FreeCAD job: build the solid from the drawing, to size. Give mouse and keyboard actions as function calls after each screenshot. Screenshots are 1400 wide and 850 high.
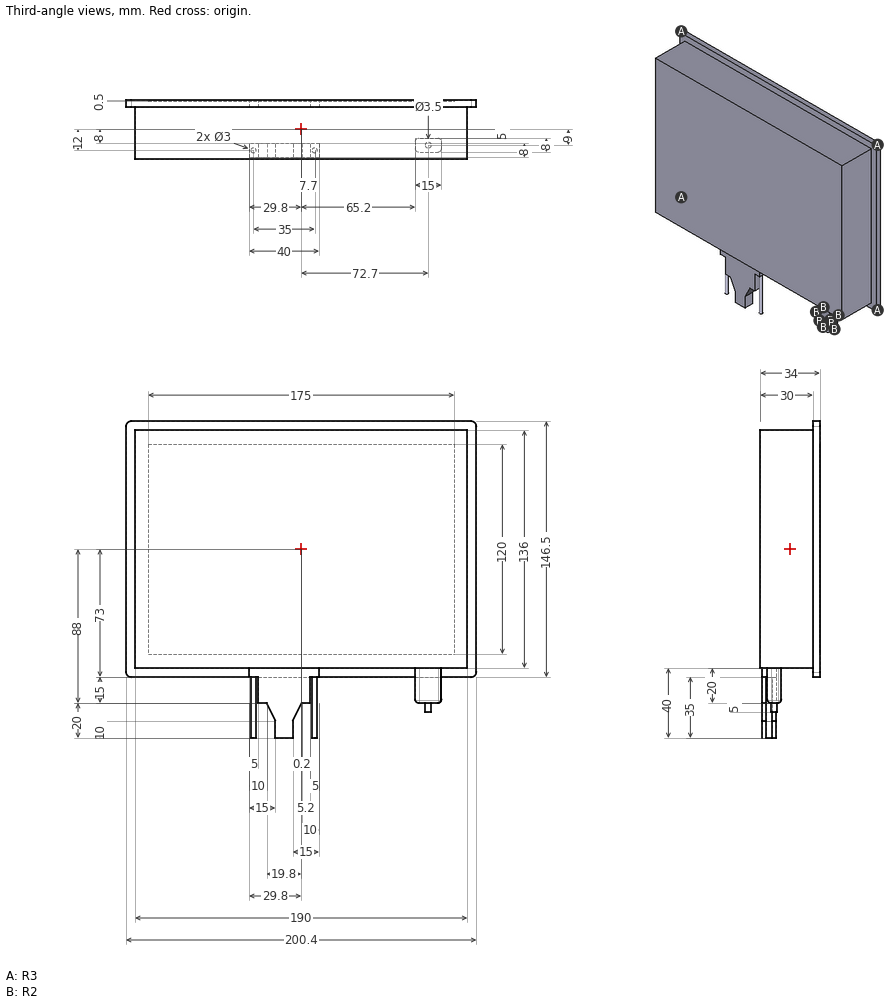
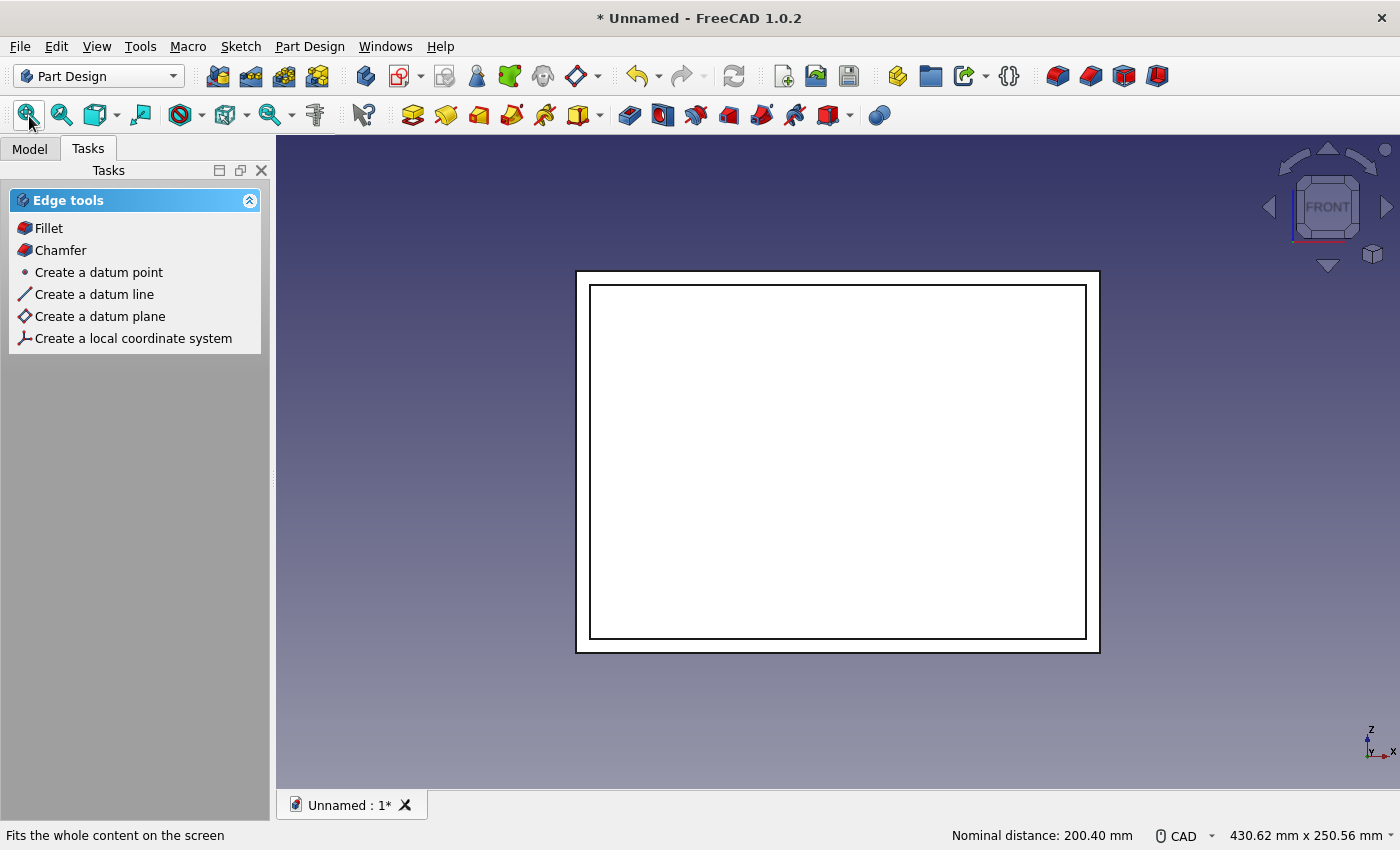
scroll(576, 652, up, 7)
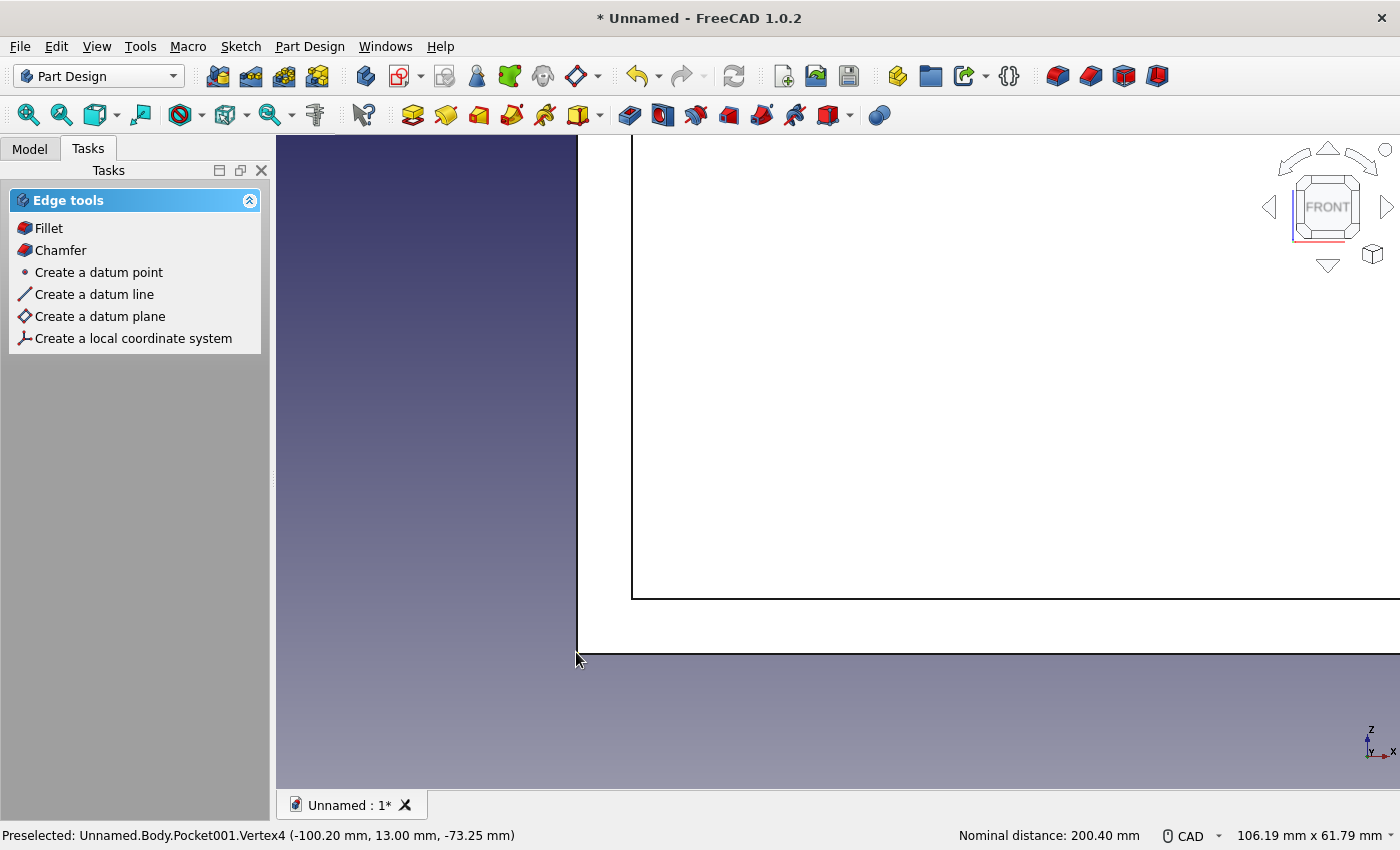
click(29, 116)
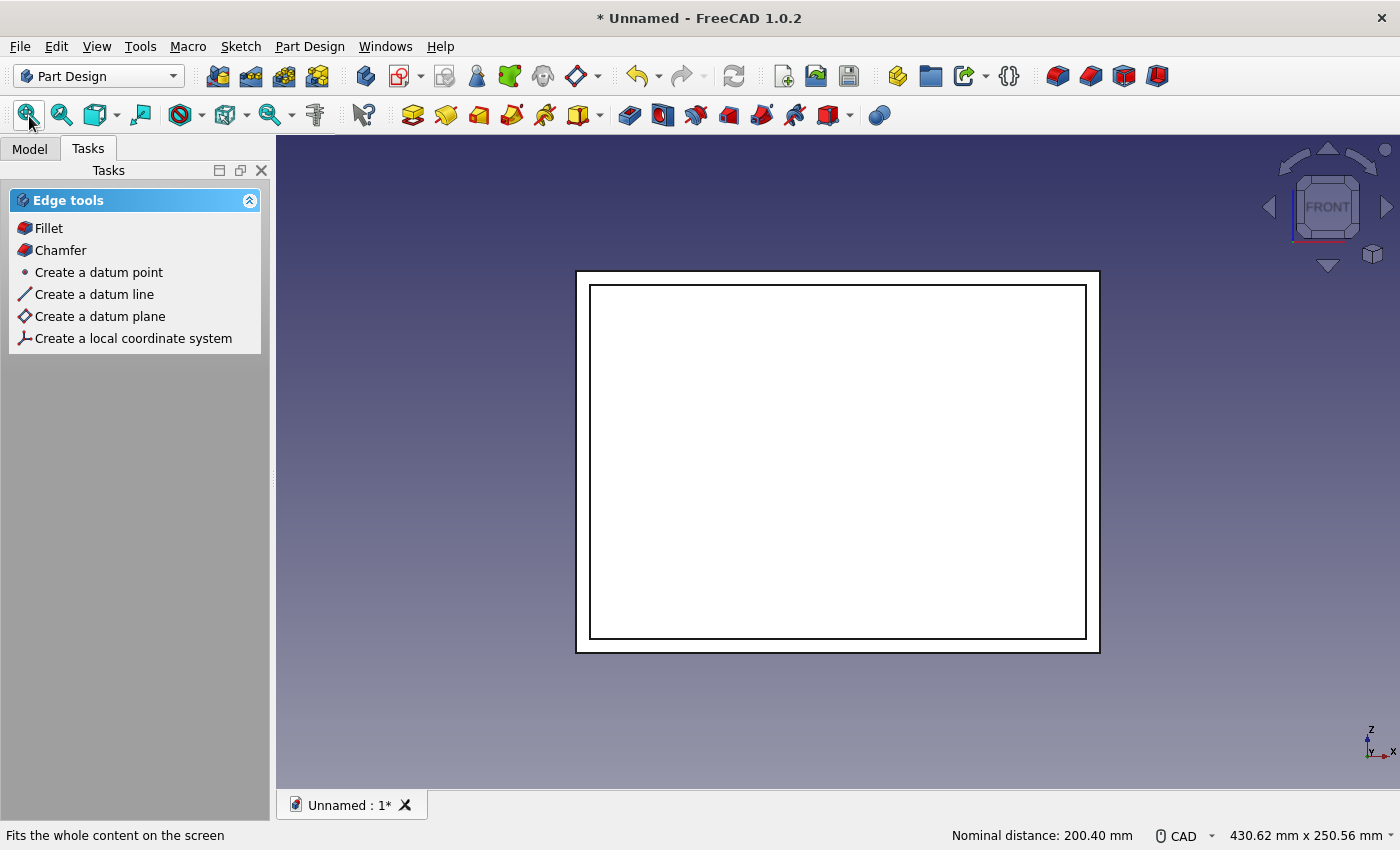
key(3)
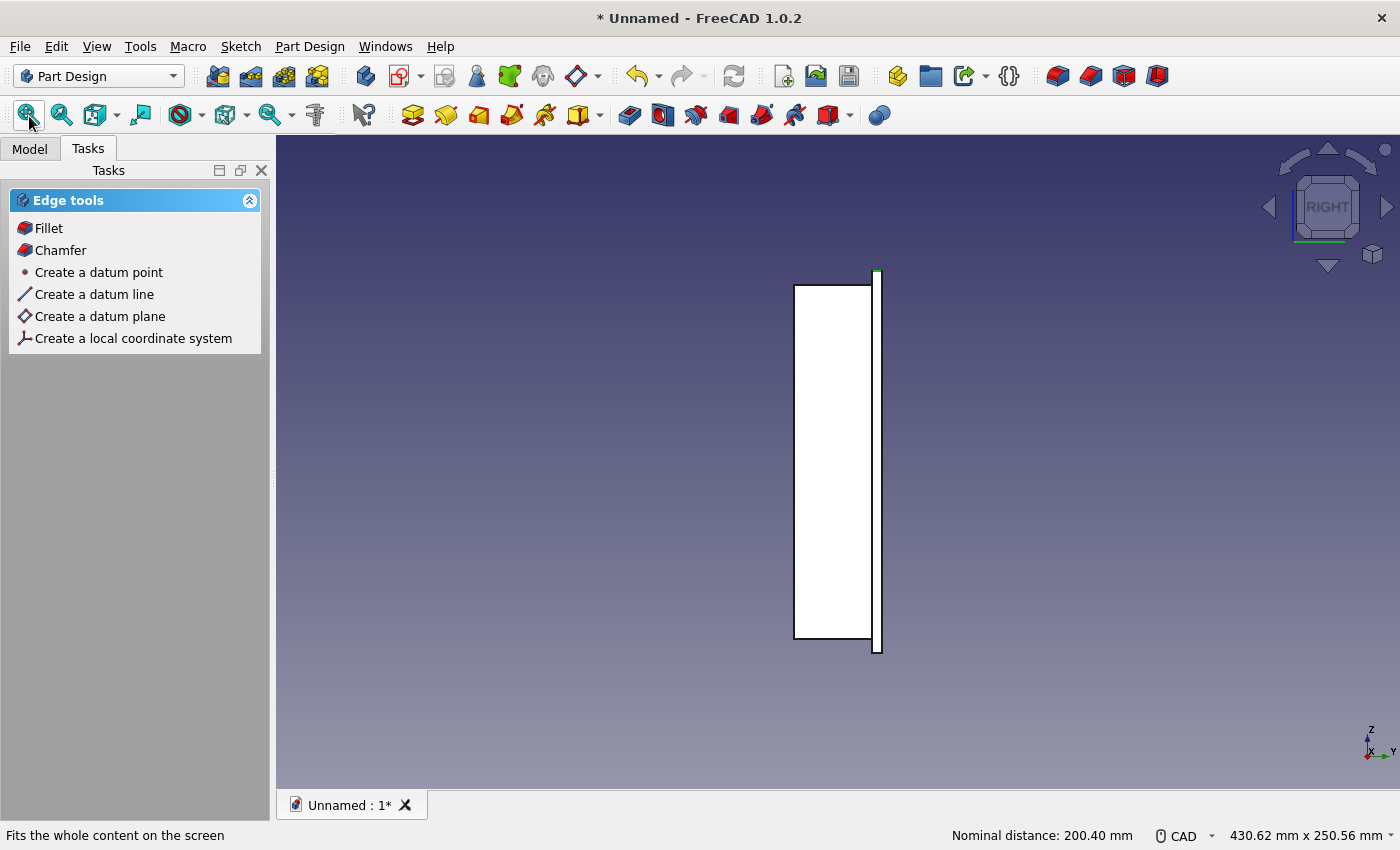
scroll(877, 652, up, 7)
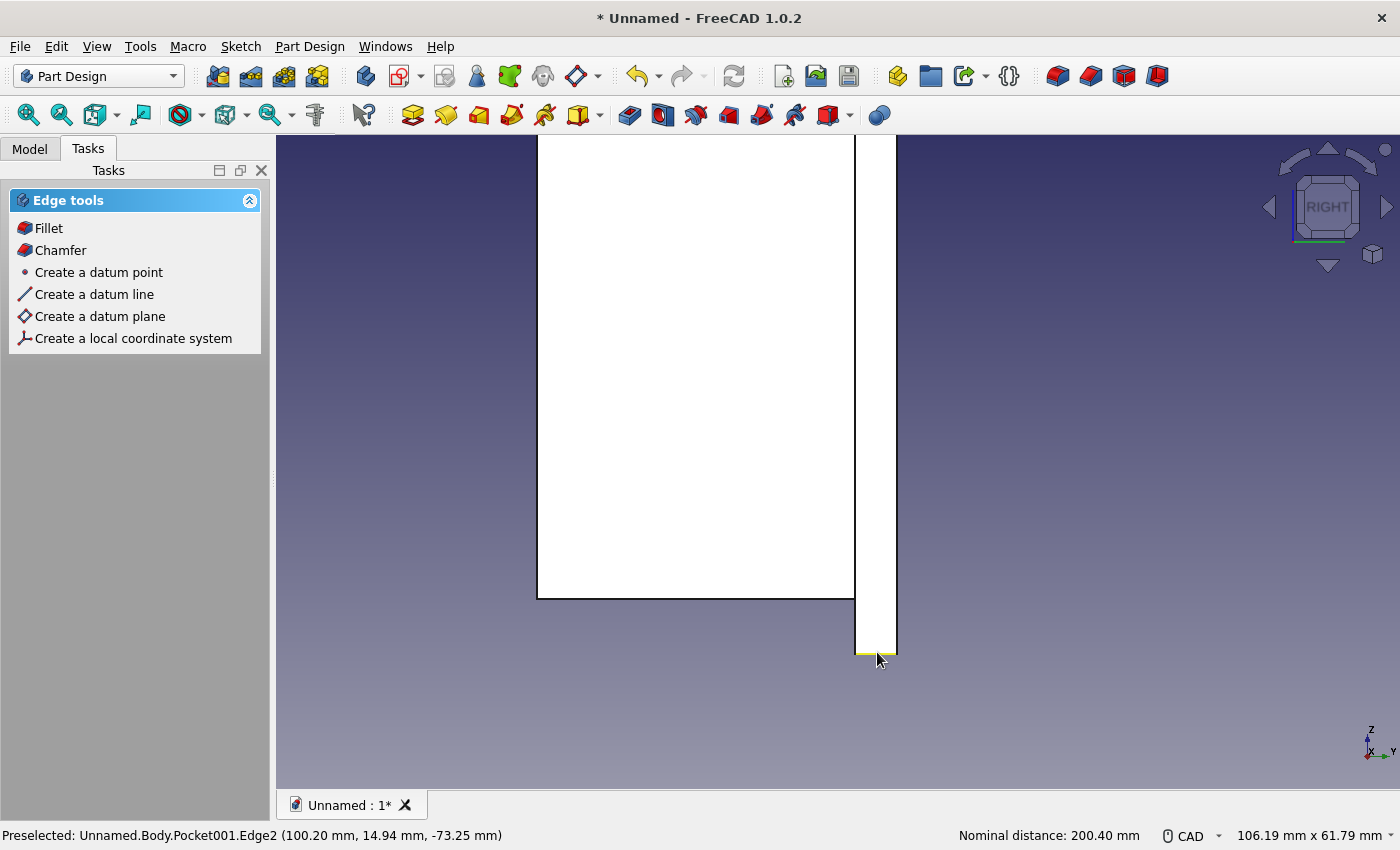
click(876, 653, ctrl)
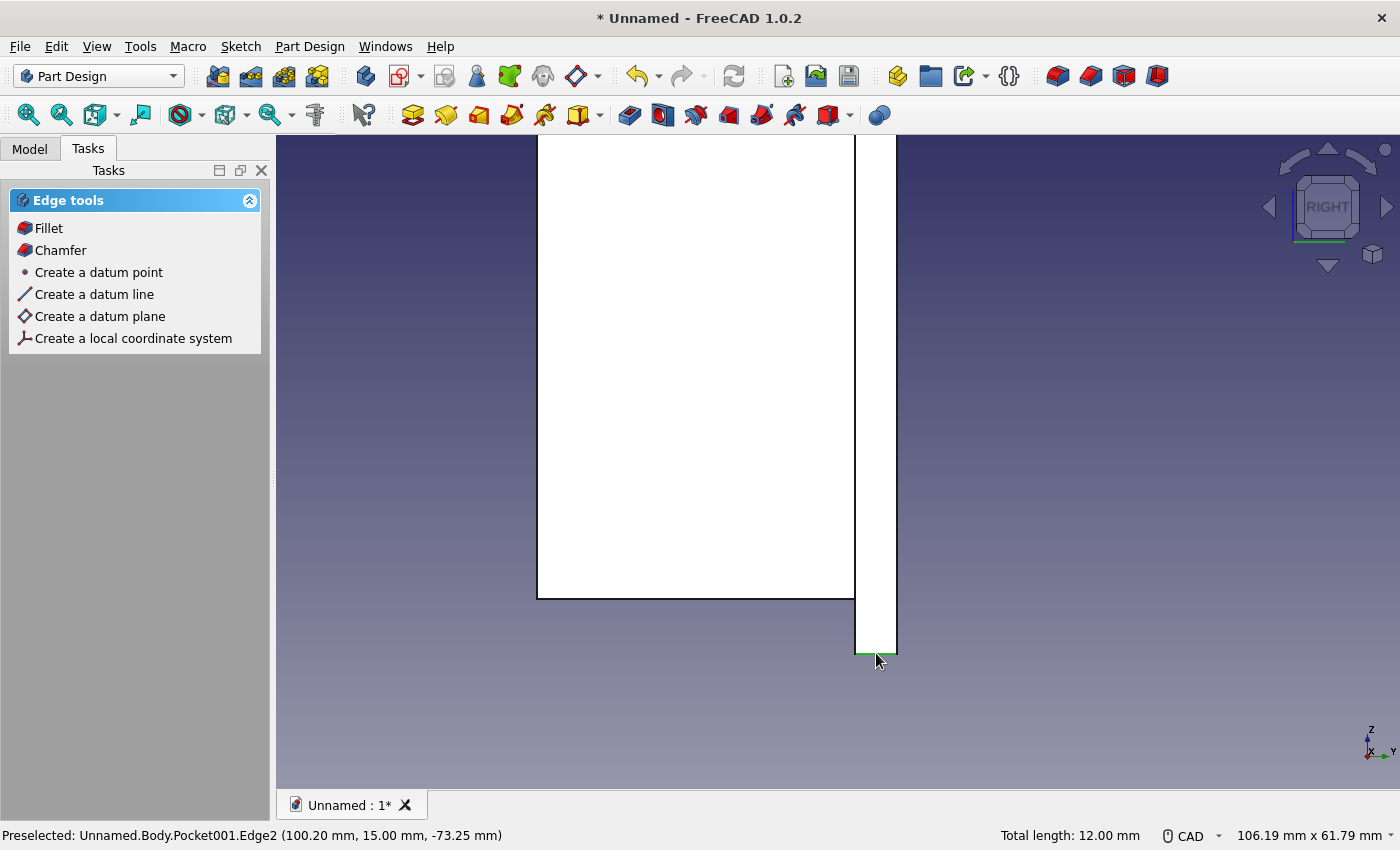
click(29, 116)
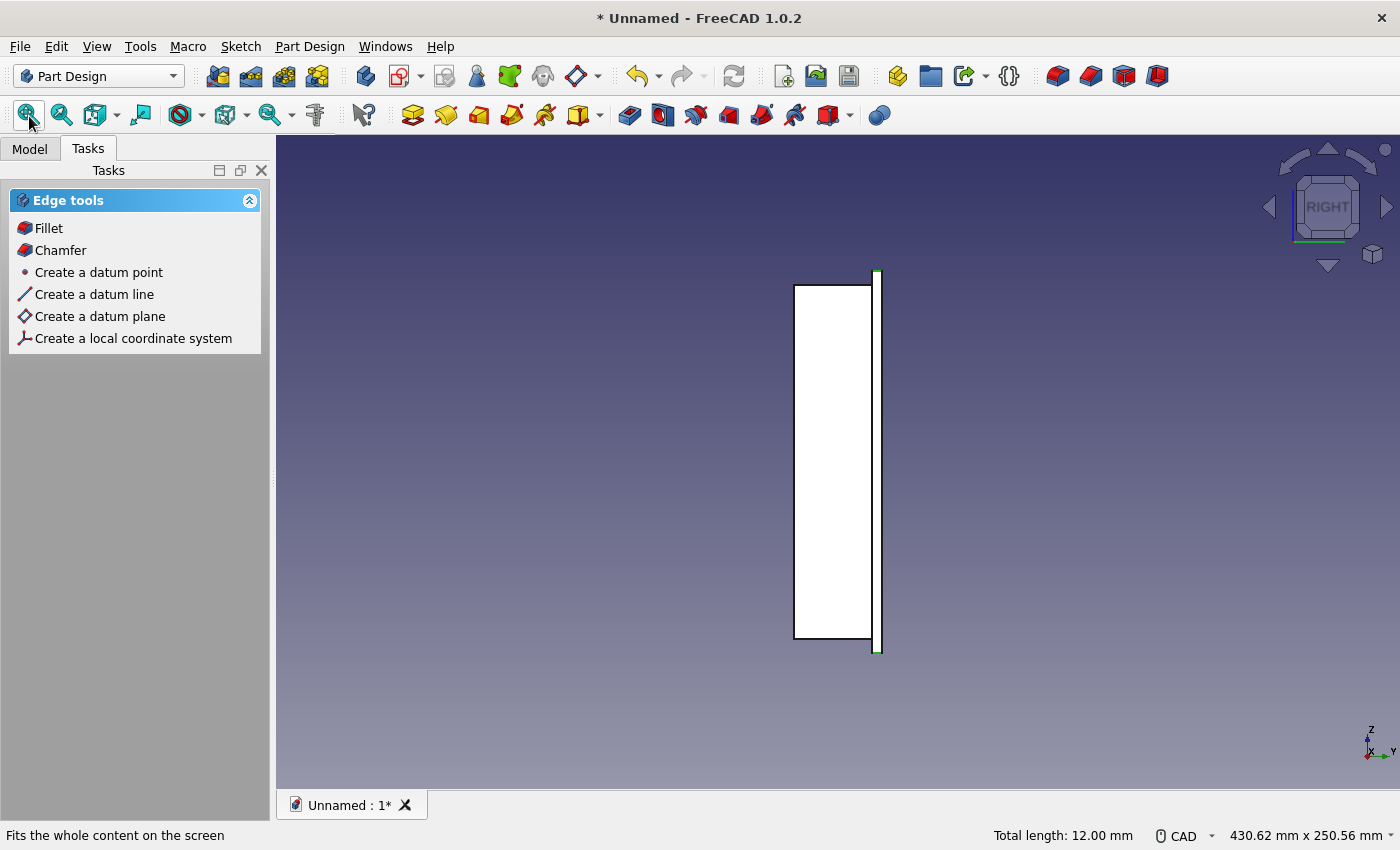
key(5)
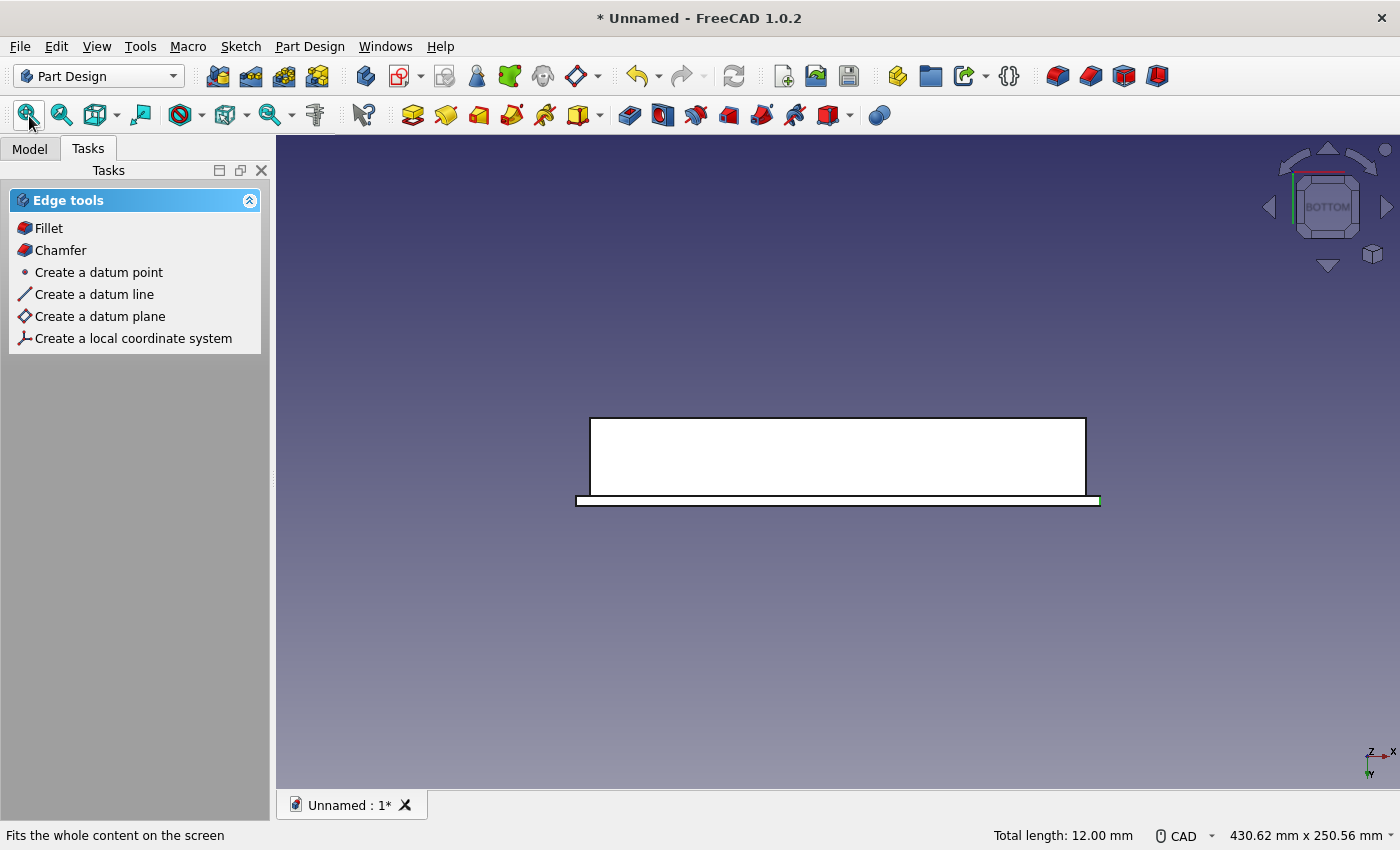
click(576, 501, ctrl)